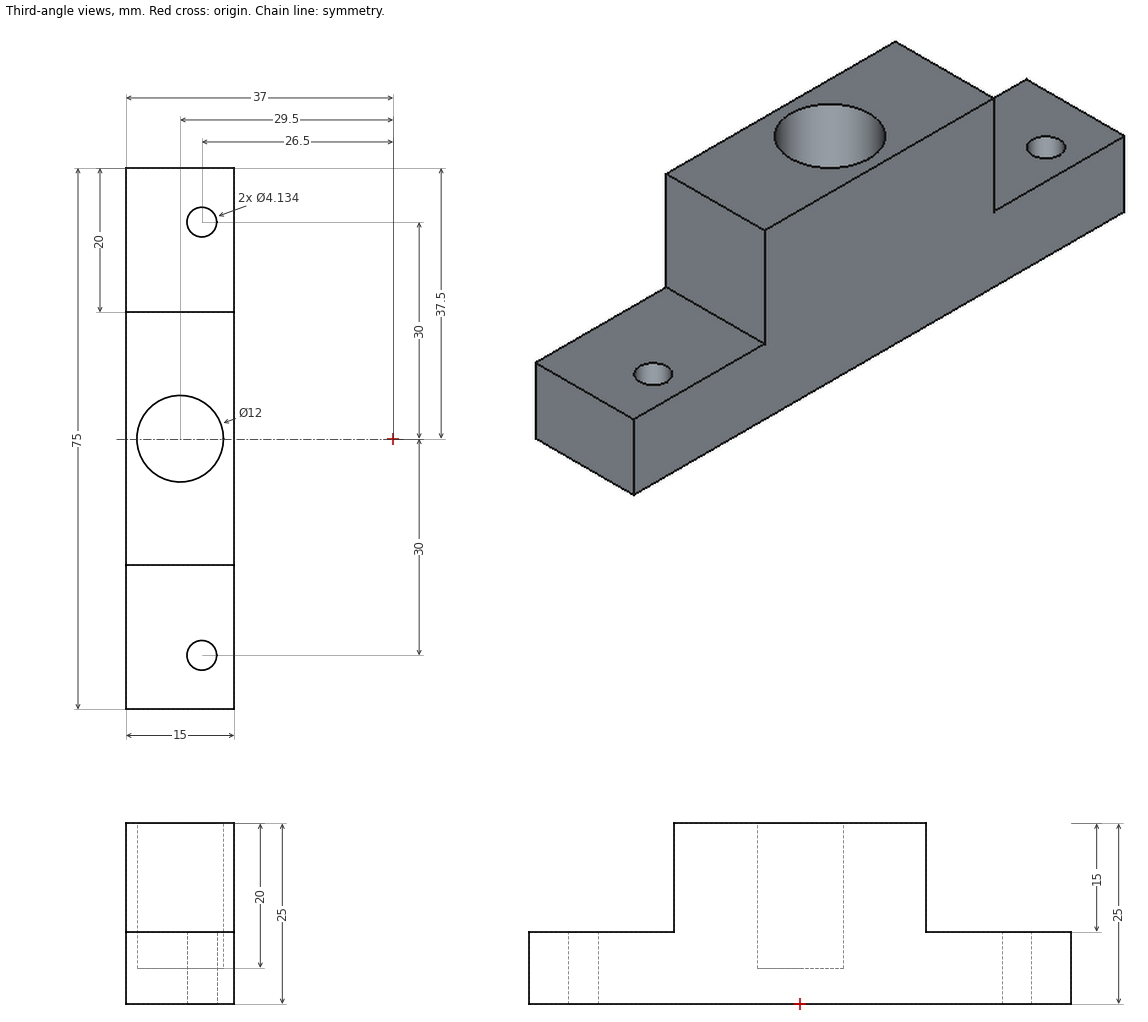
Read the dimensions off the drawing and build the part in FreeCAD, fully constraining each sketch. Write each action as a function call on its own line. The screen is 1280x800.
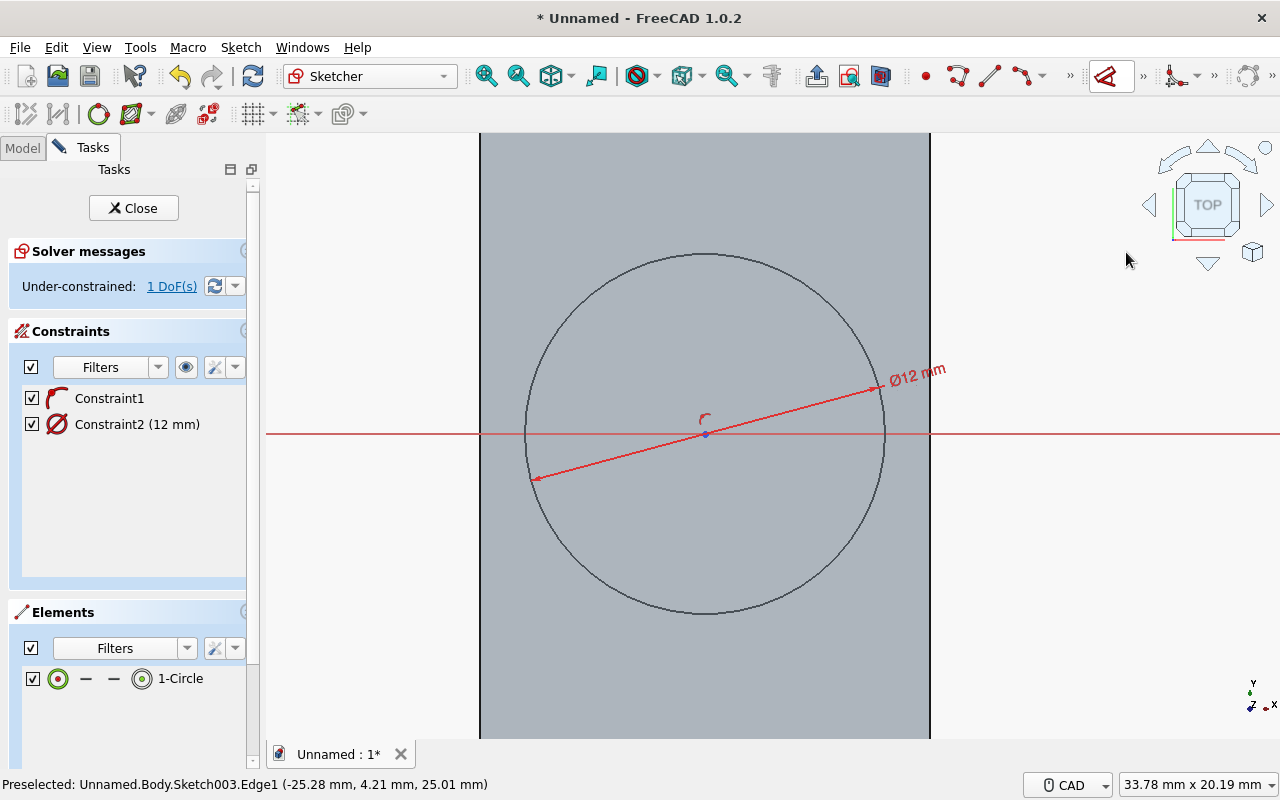
click(705, 434)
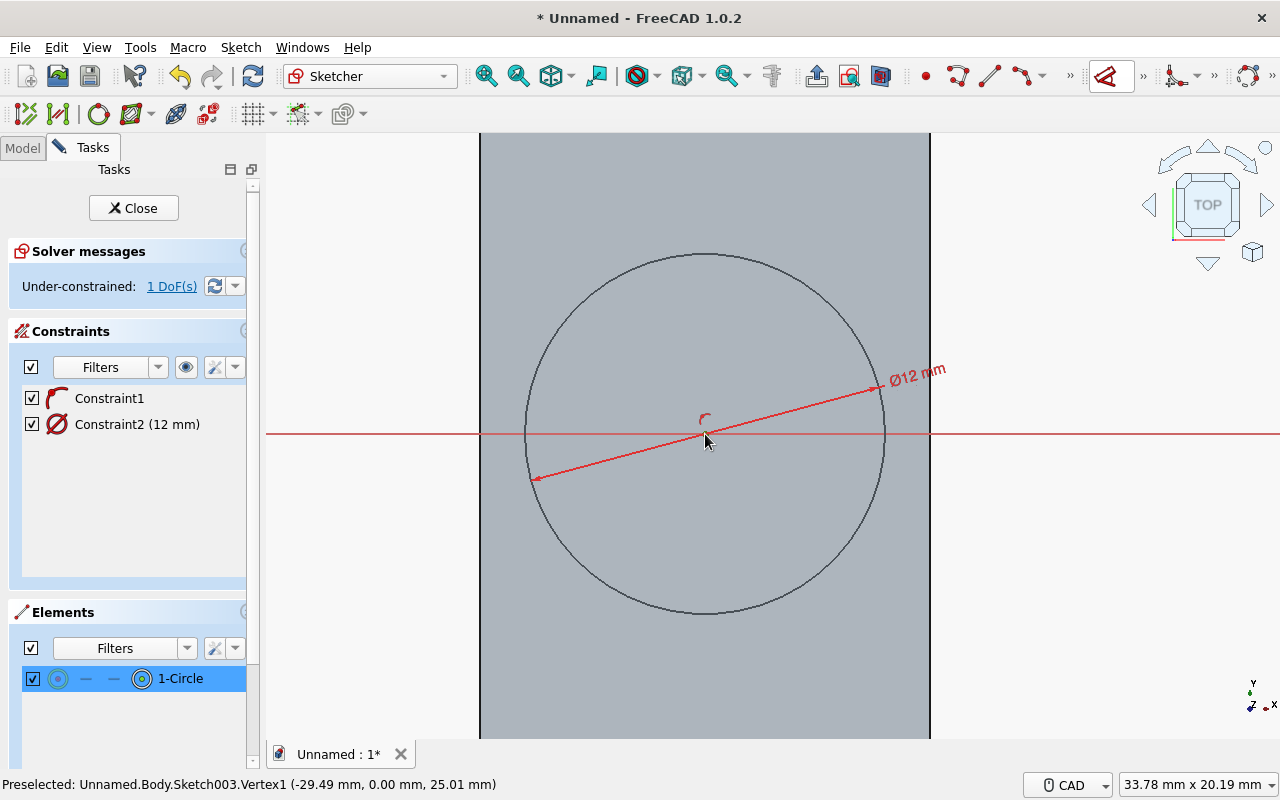
click(1128, 76)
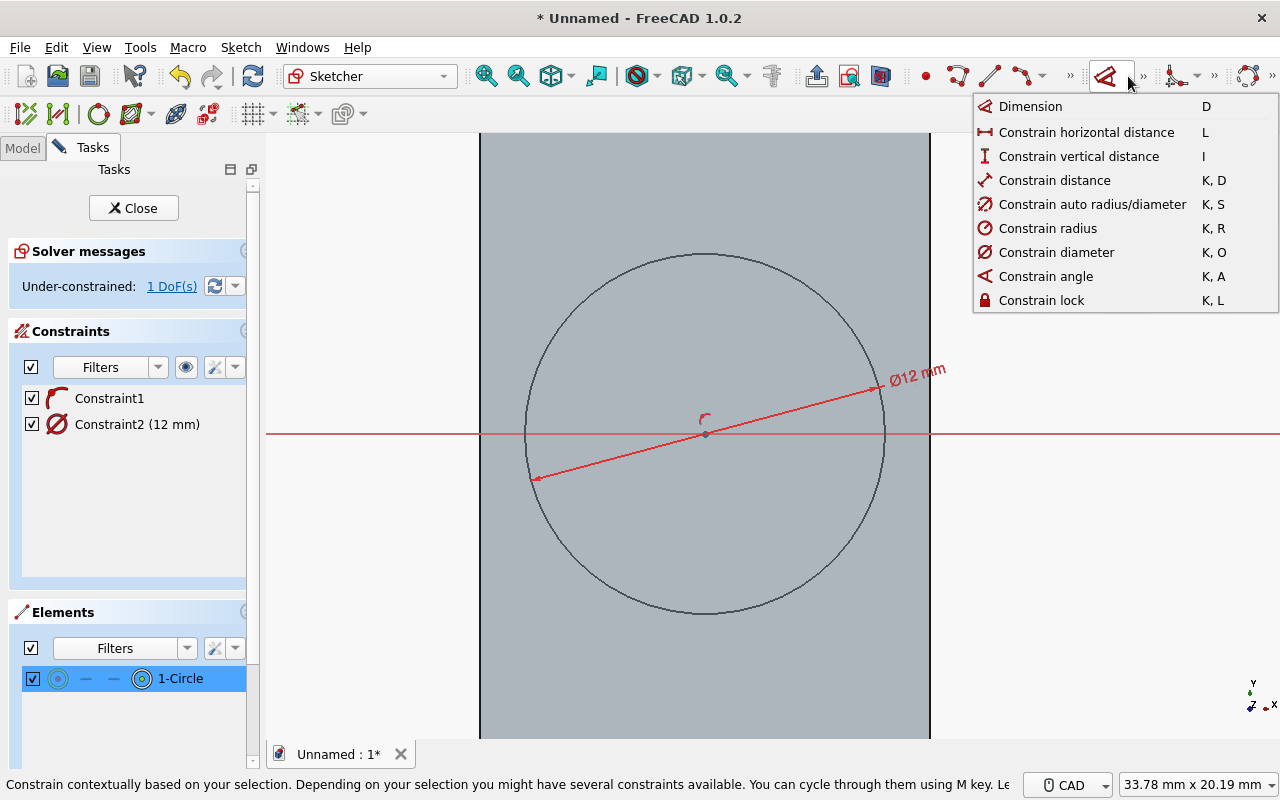
click(1126, 132)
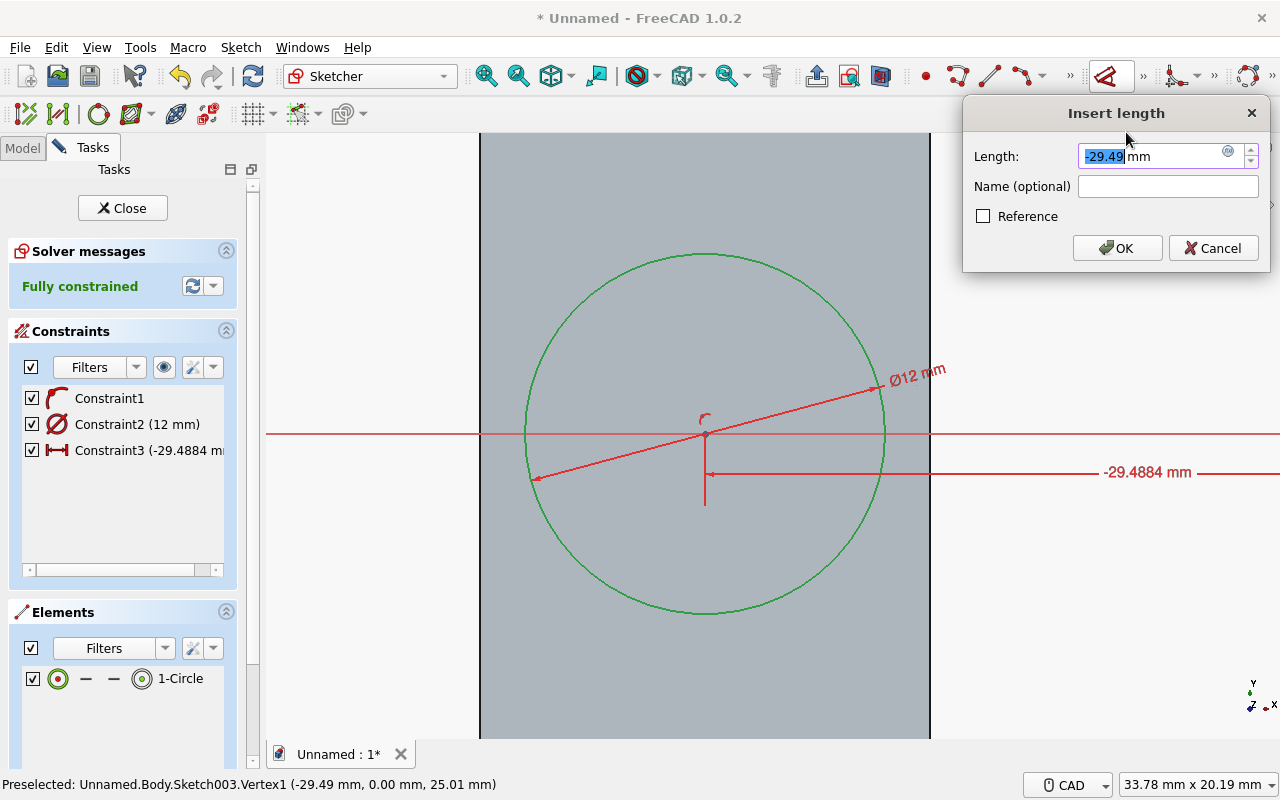
text(-29.5)
key(Return)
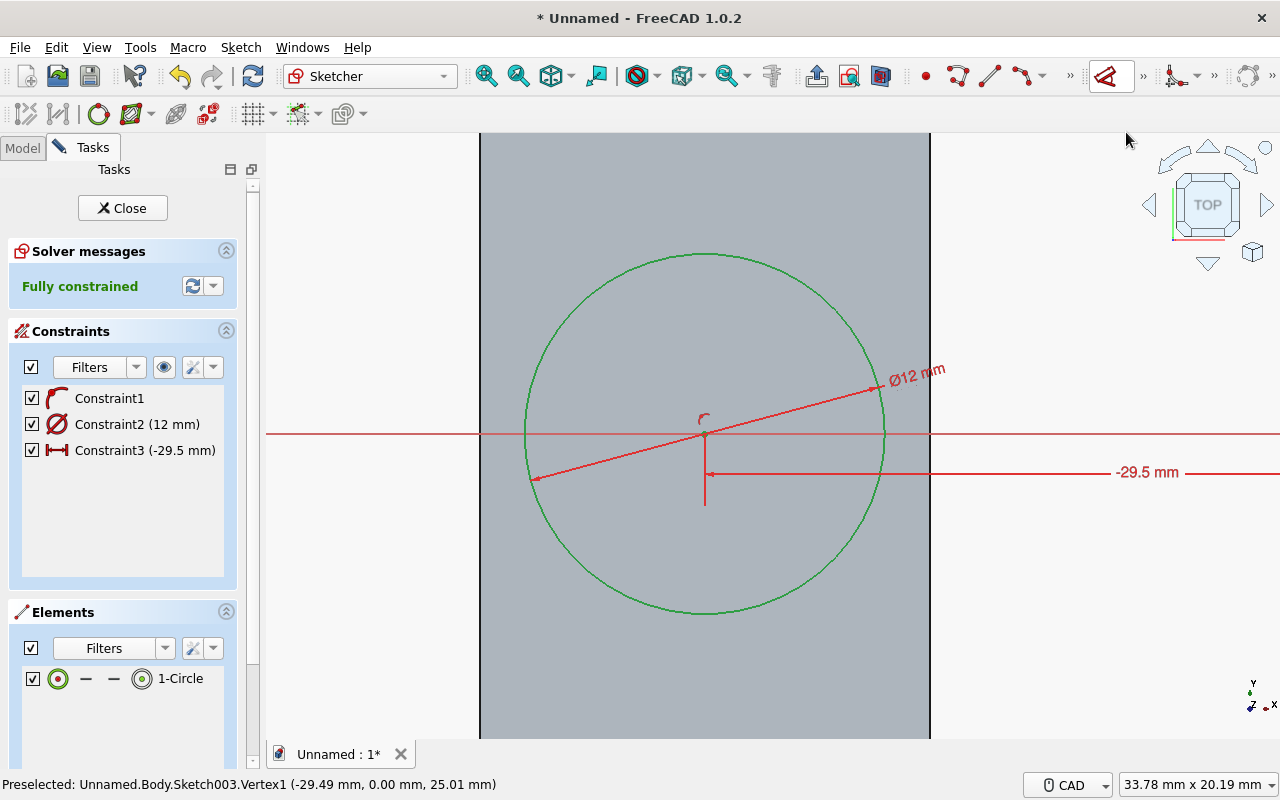
click(123, 208)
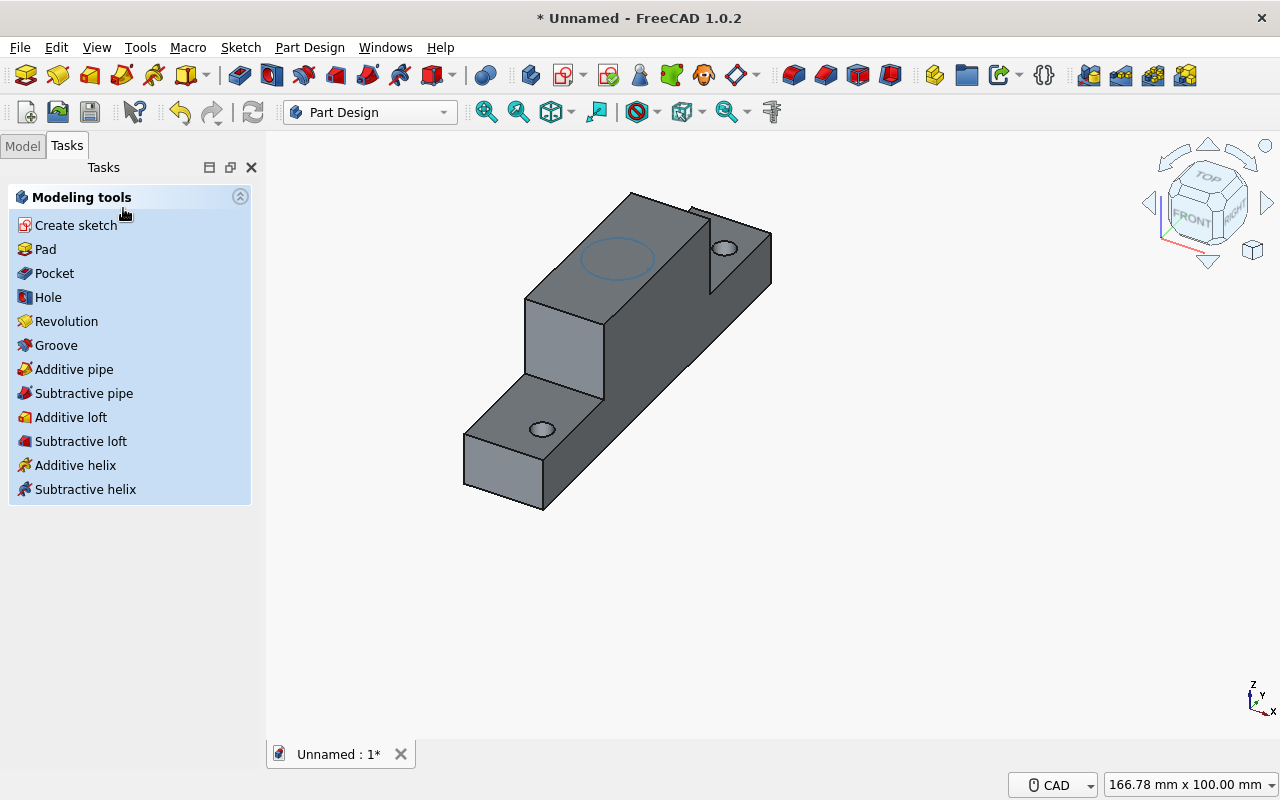
click(240, 76)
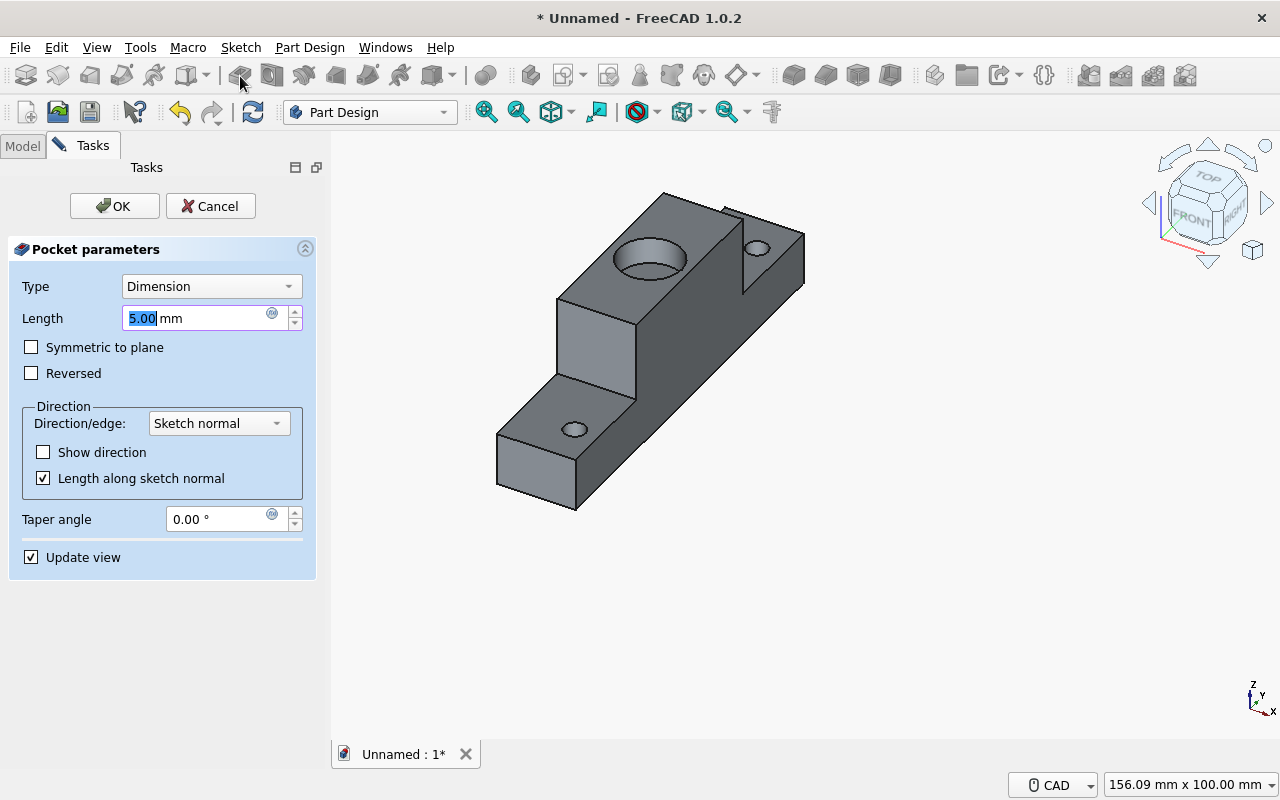
text(20)
key(Tab)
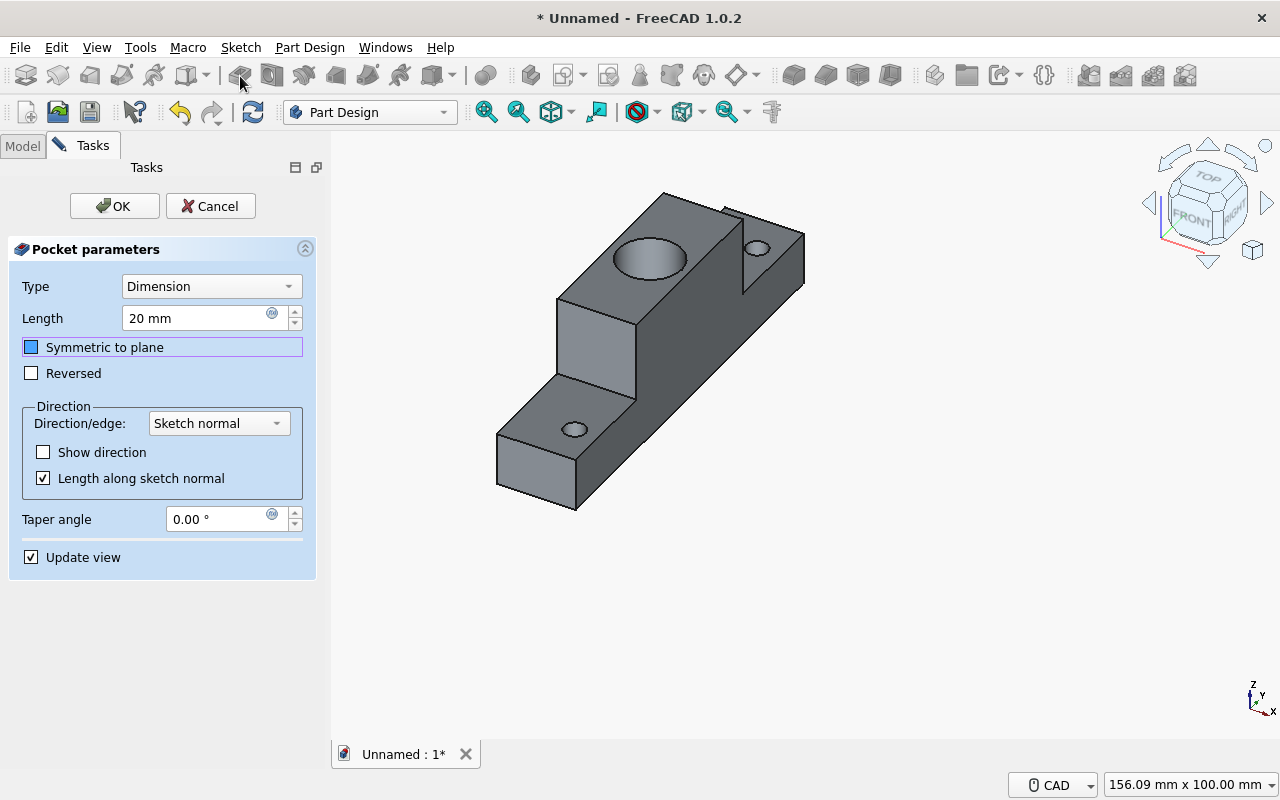
click(115, 206)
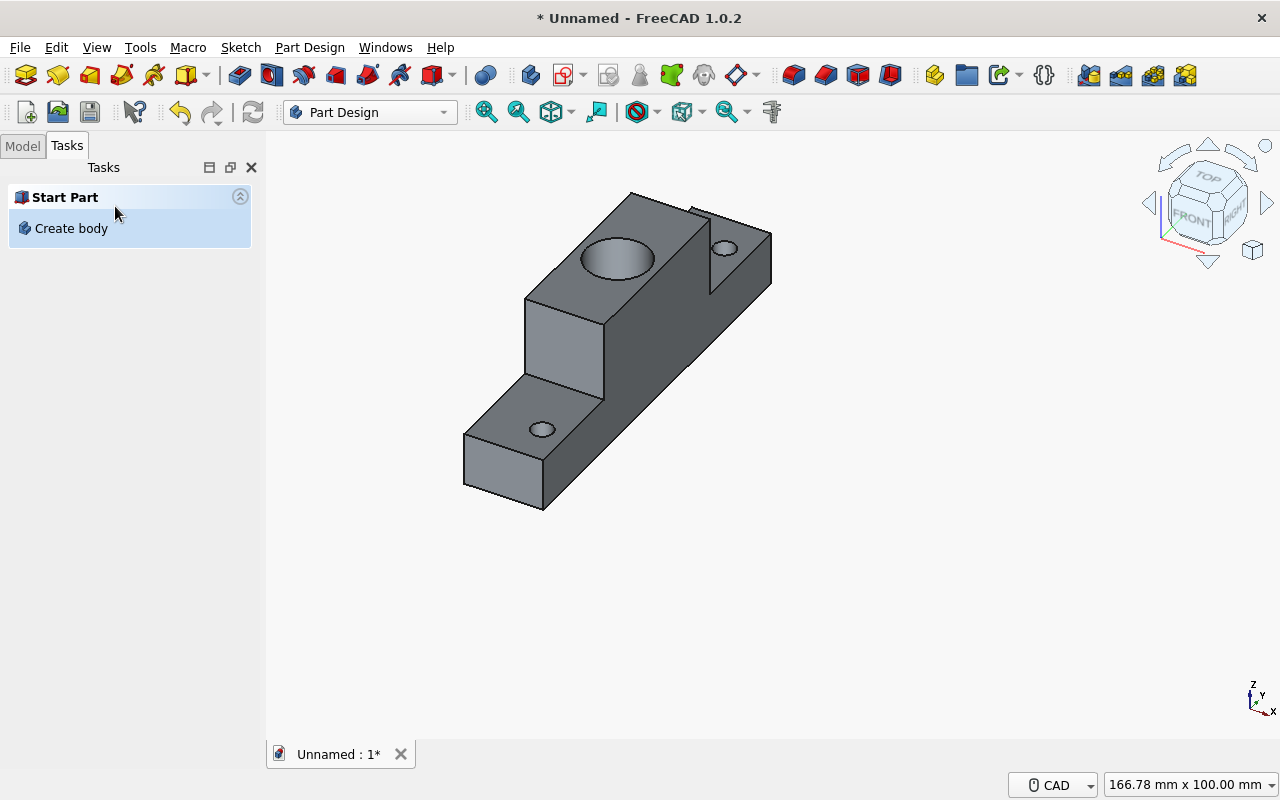
key(0)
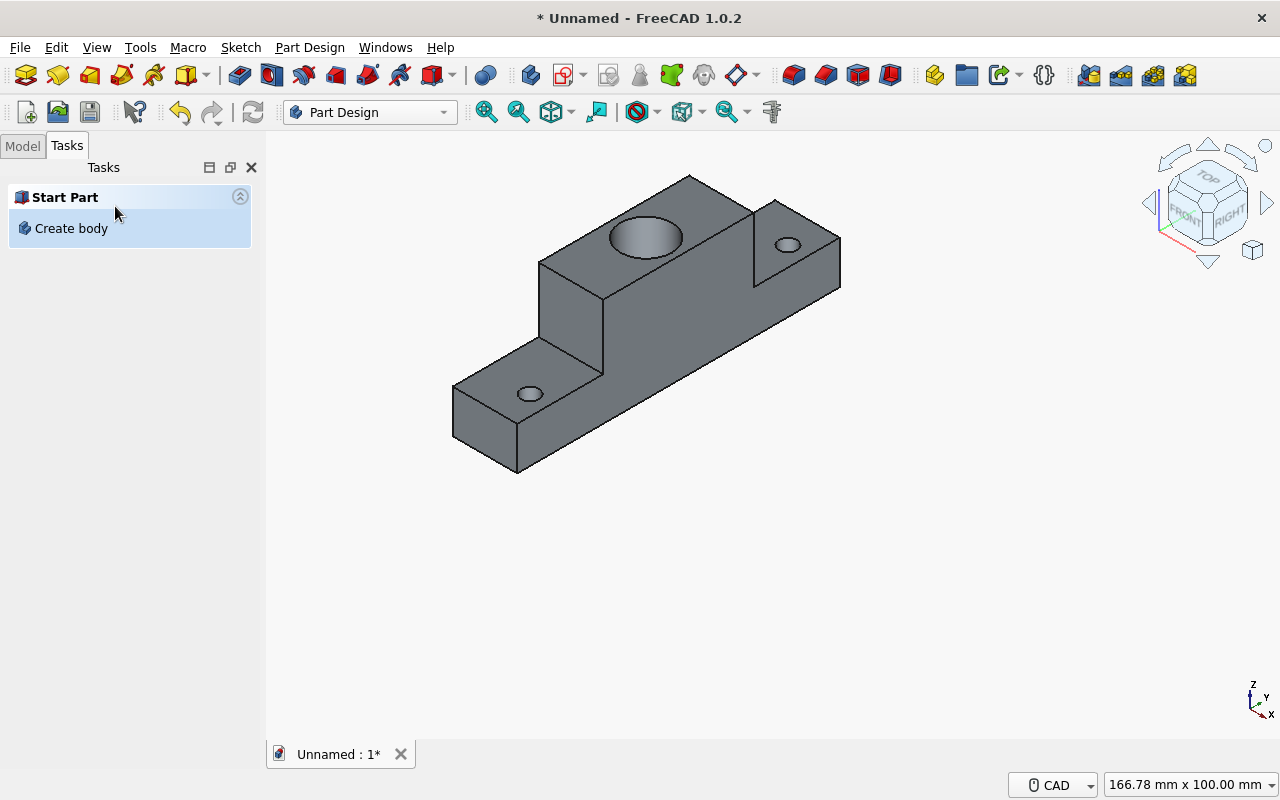
click(488, 112)